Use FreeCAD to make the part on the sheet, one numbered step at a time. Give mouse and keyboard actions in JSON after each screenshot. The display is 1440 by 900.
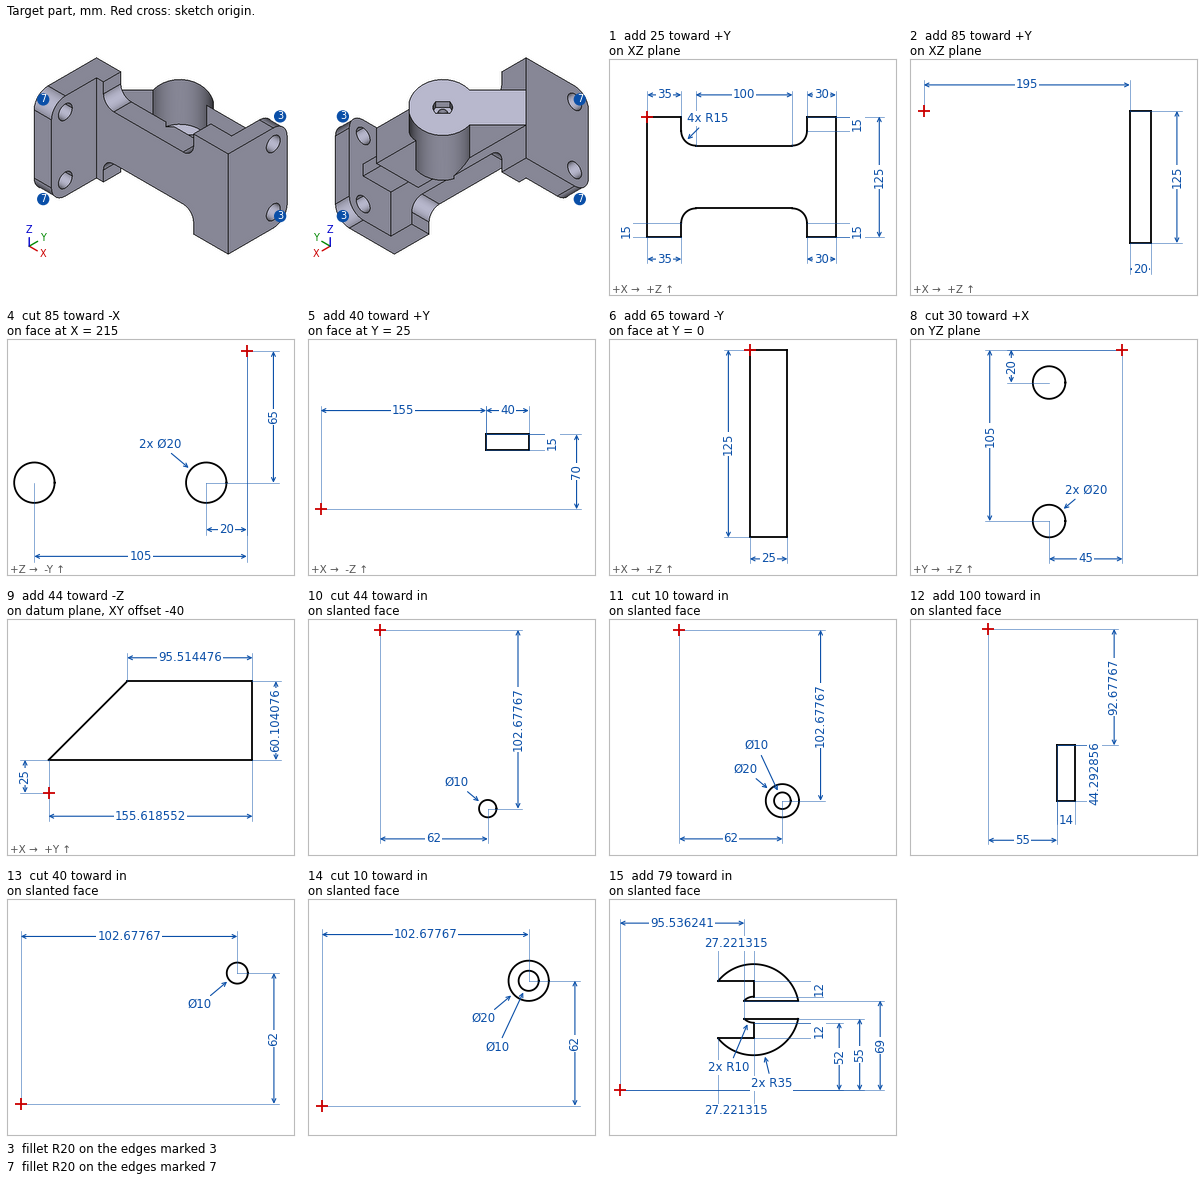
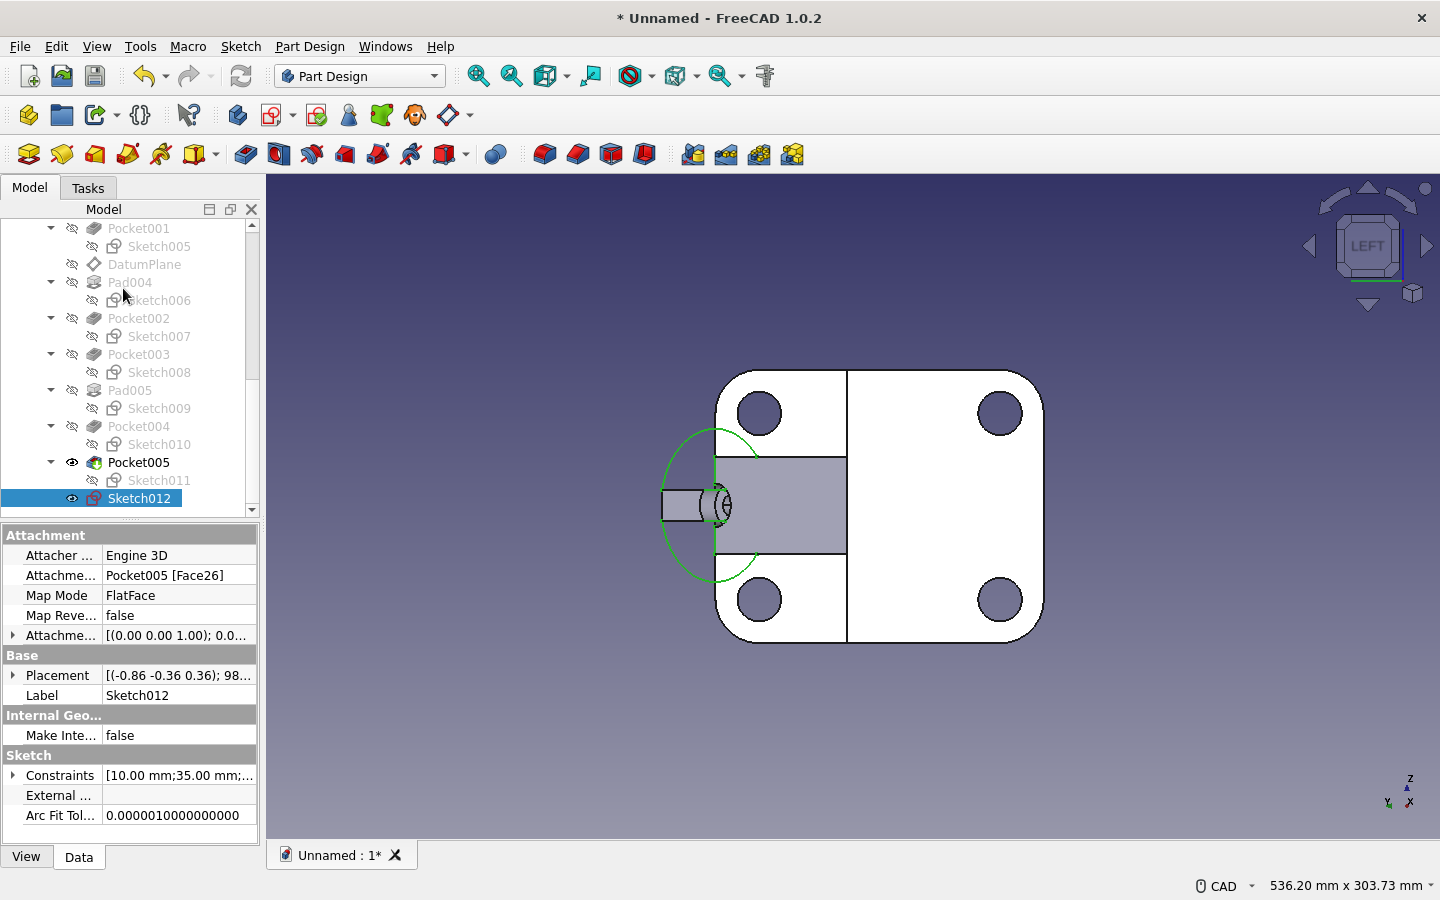
{"action": "left_click", "coordinate": [29, 154]}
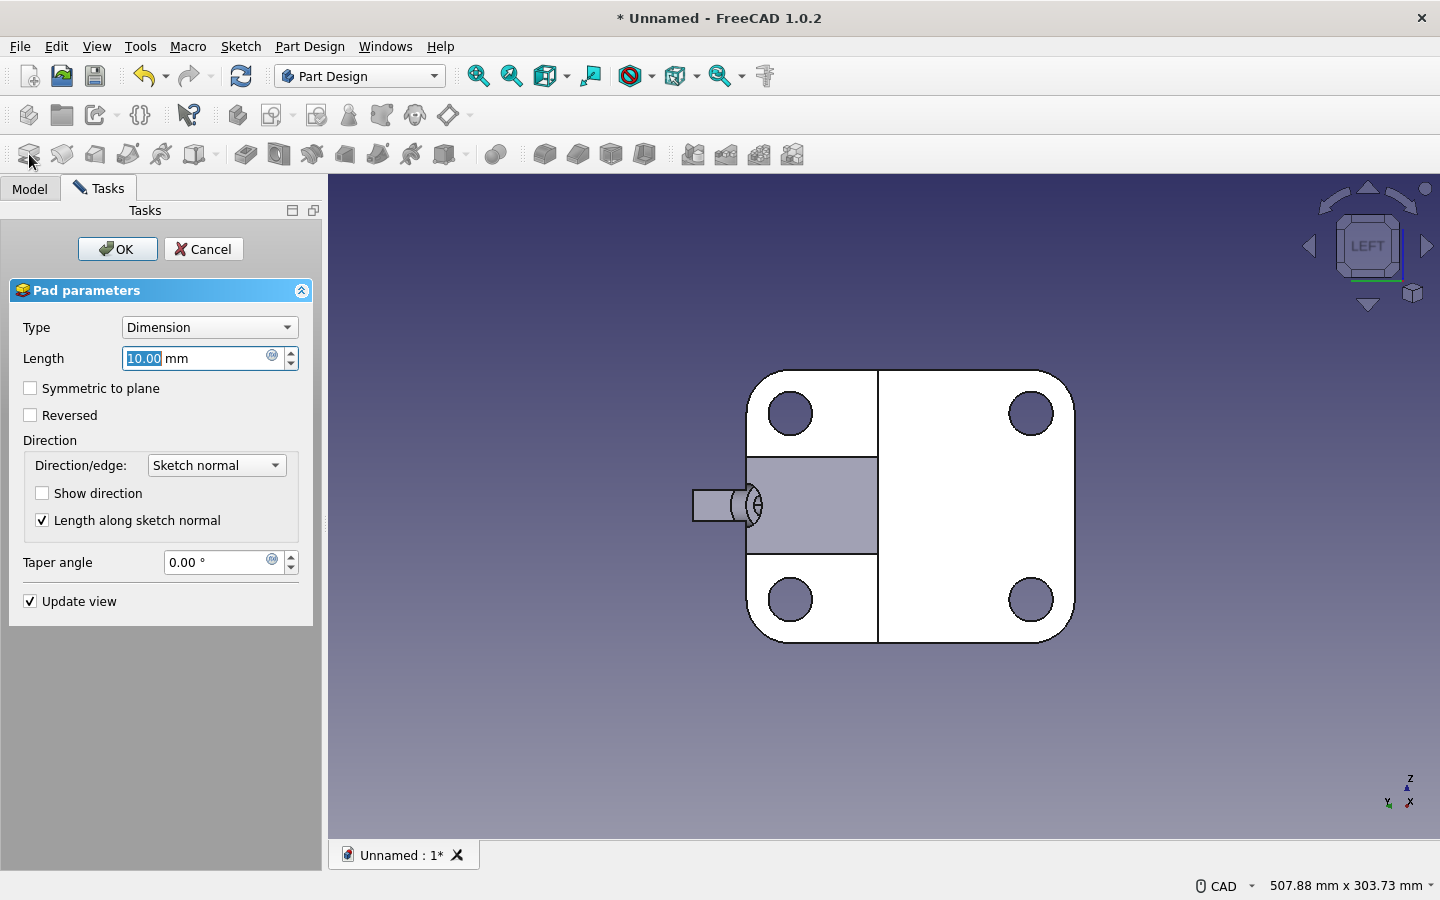
{"action": "type", "text": "79"}
{"action": "key", "text": "Tab"}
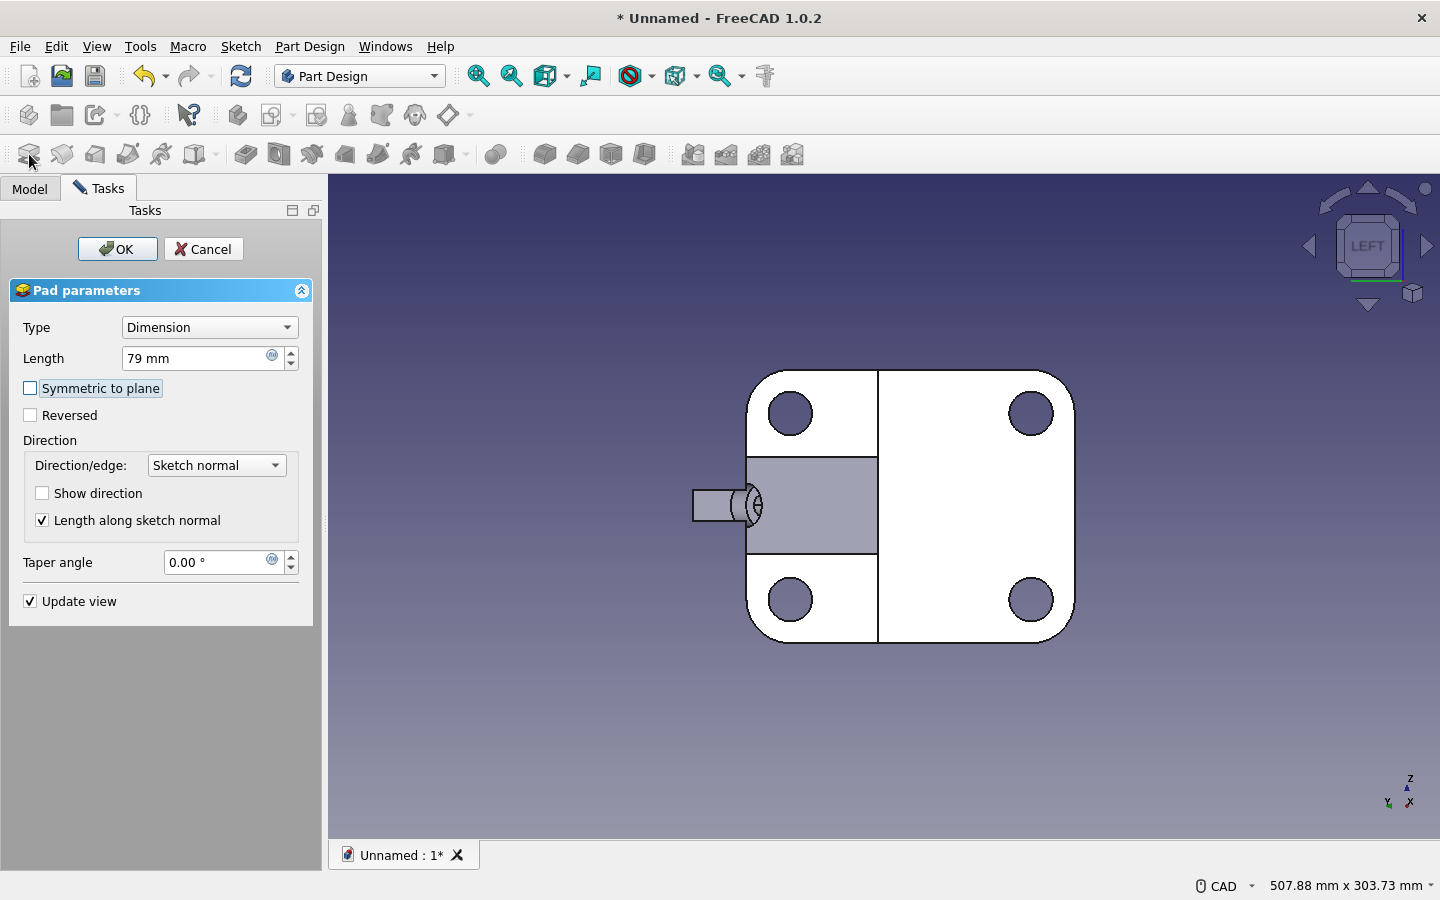
{"action": "left_click", "coordinate": [31, 415]}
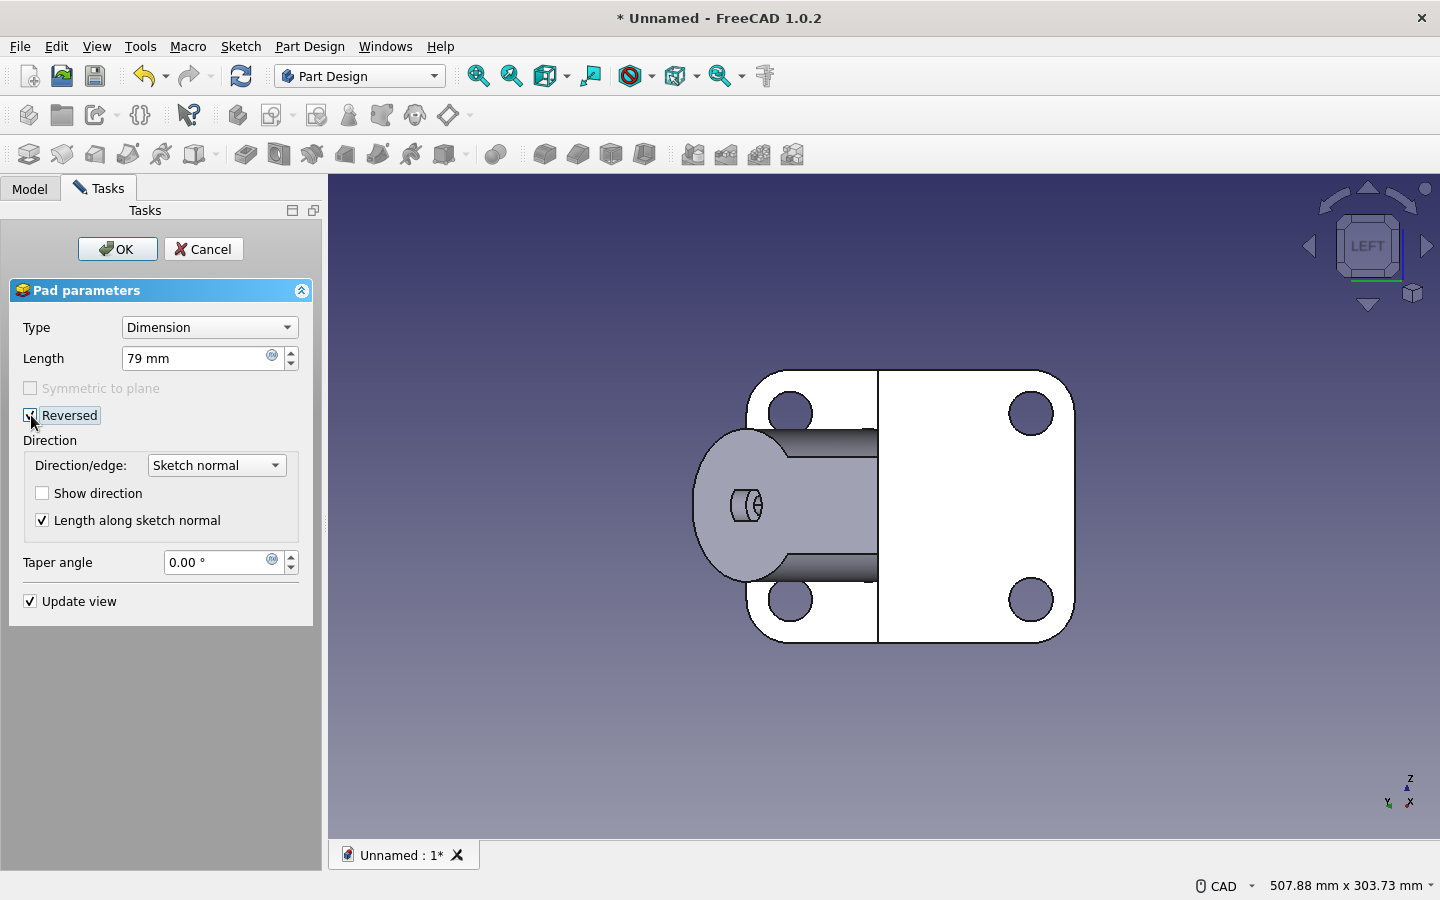
{"action": "left_click", "coordinate": [118, 249]}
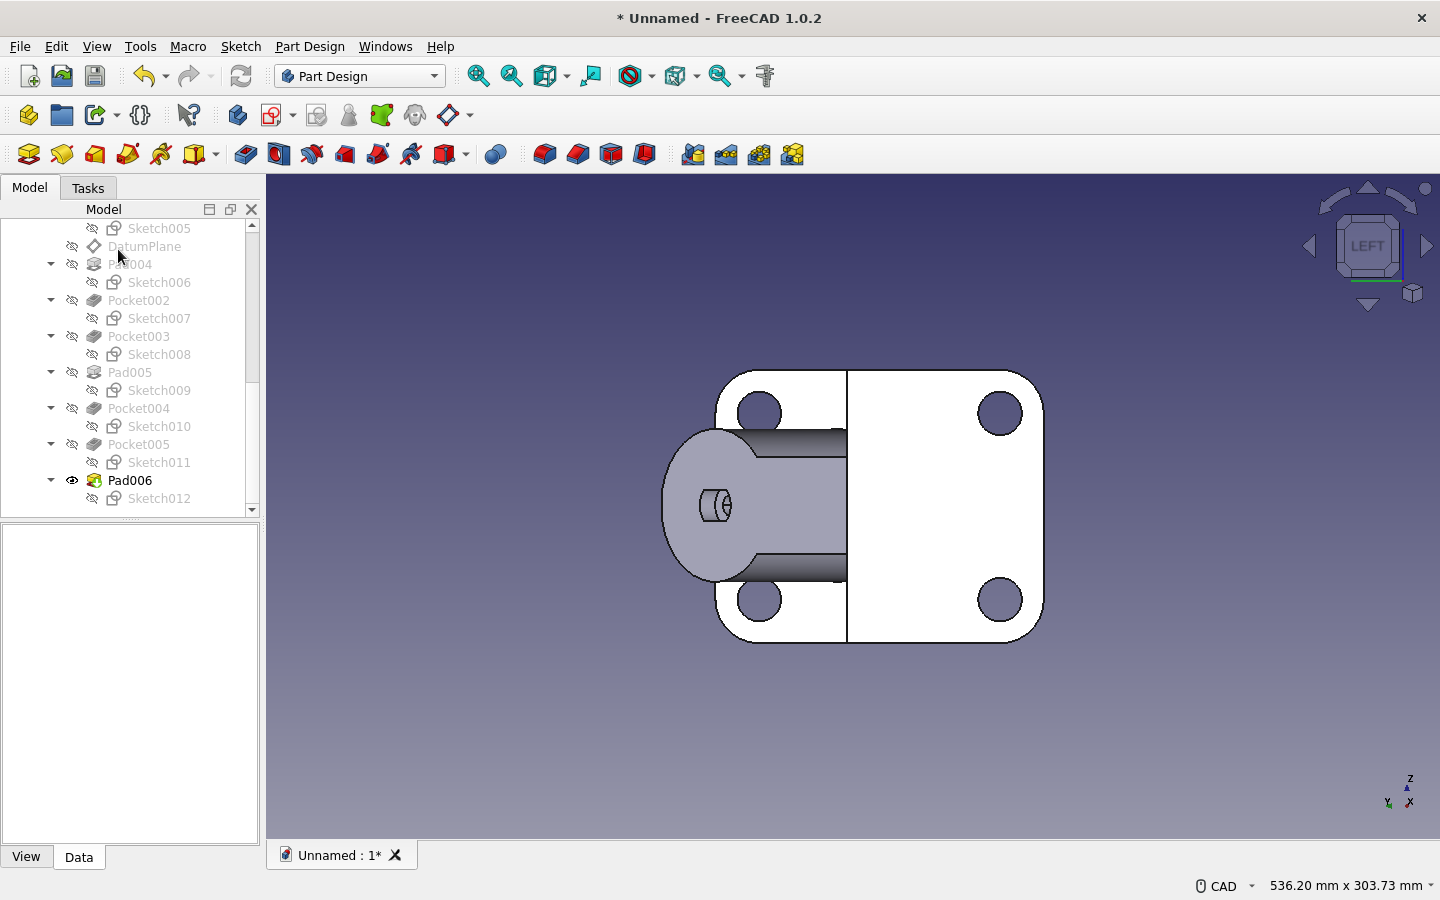
{"action": "key", "text": "0"}